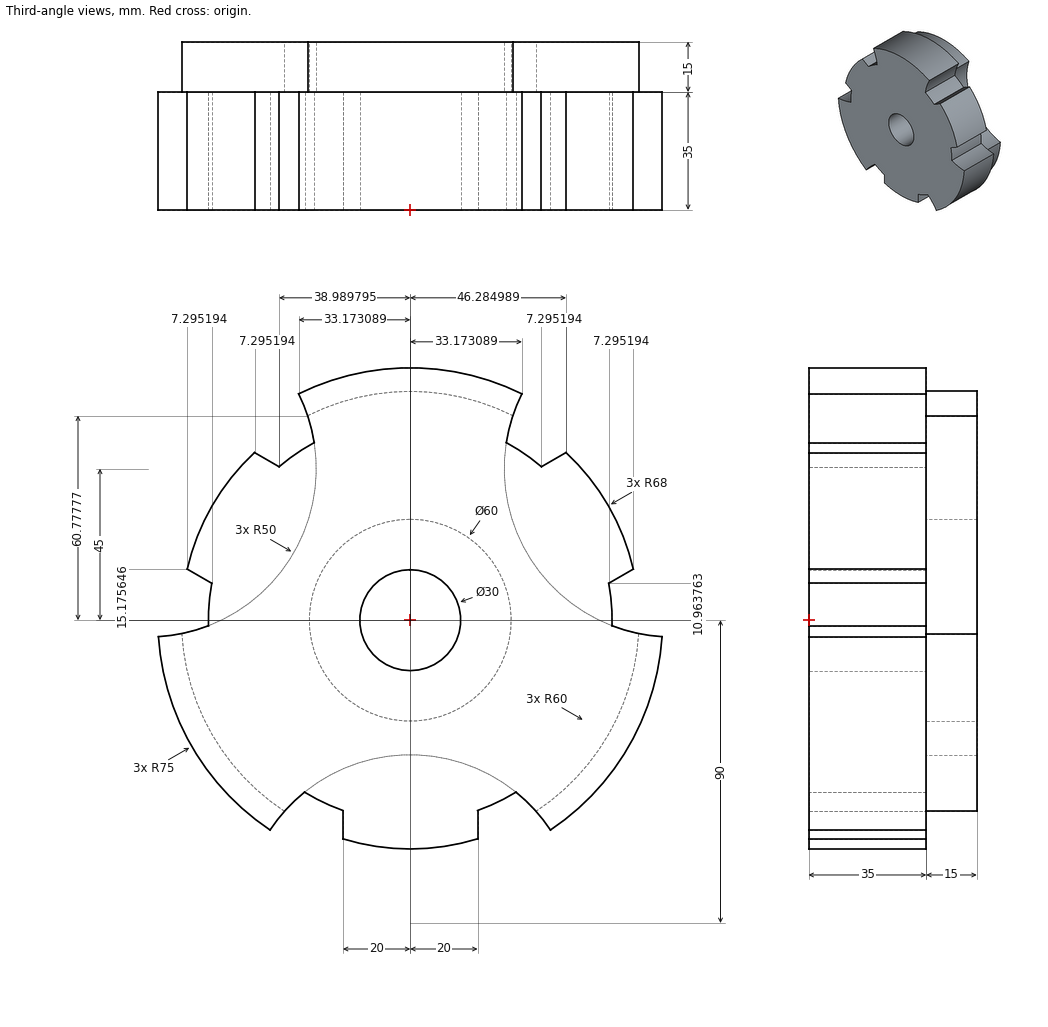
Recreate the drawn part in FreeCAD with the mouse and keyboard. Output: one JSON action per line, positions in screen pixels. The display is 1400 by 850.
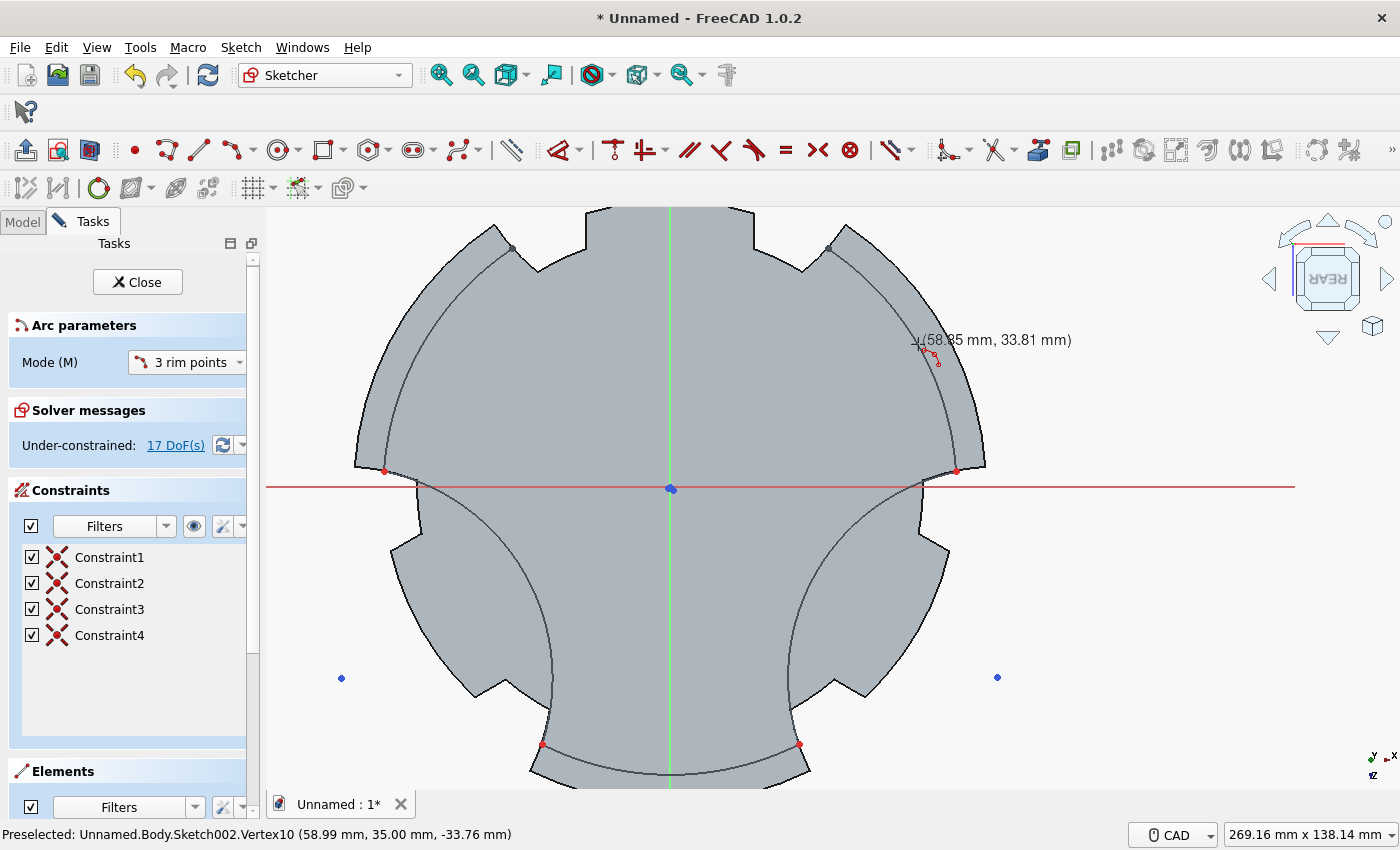
{"action": "left_click", "coordinate": [828, 249]}
{"action": "left_click", "coordinate": [512, 249]}
{"action": "left_click", "coordinate": [635, 316]}
{"action": "key", "text": "Escape"}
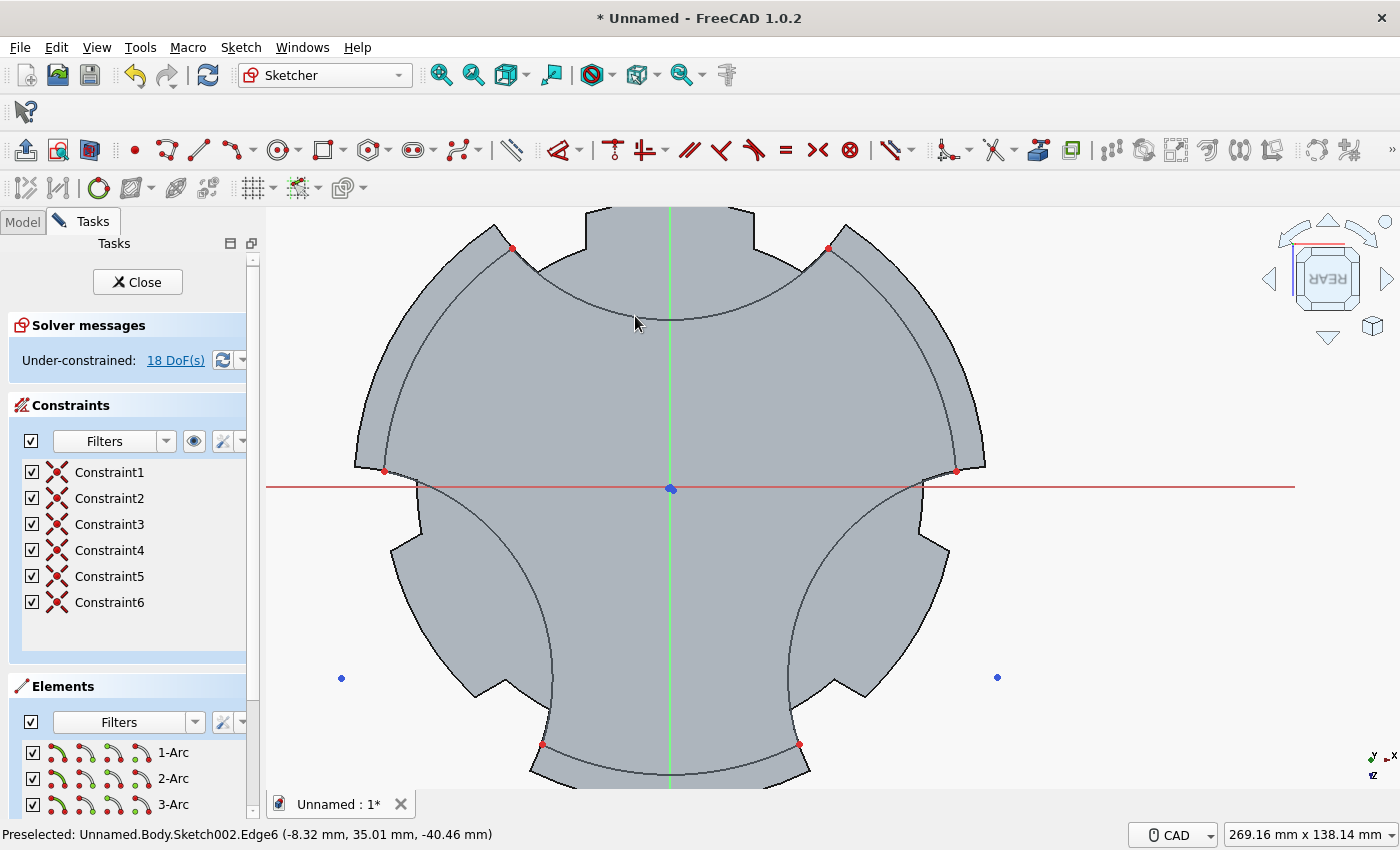
{"action": "left_click", "coordinate": [453, 302]}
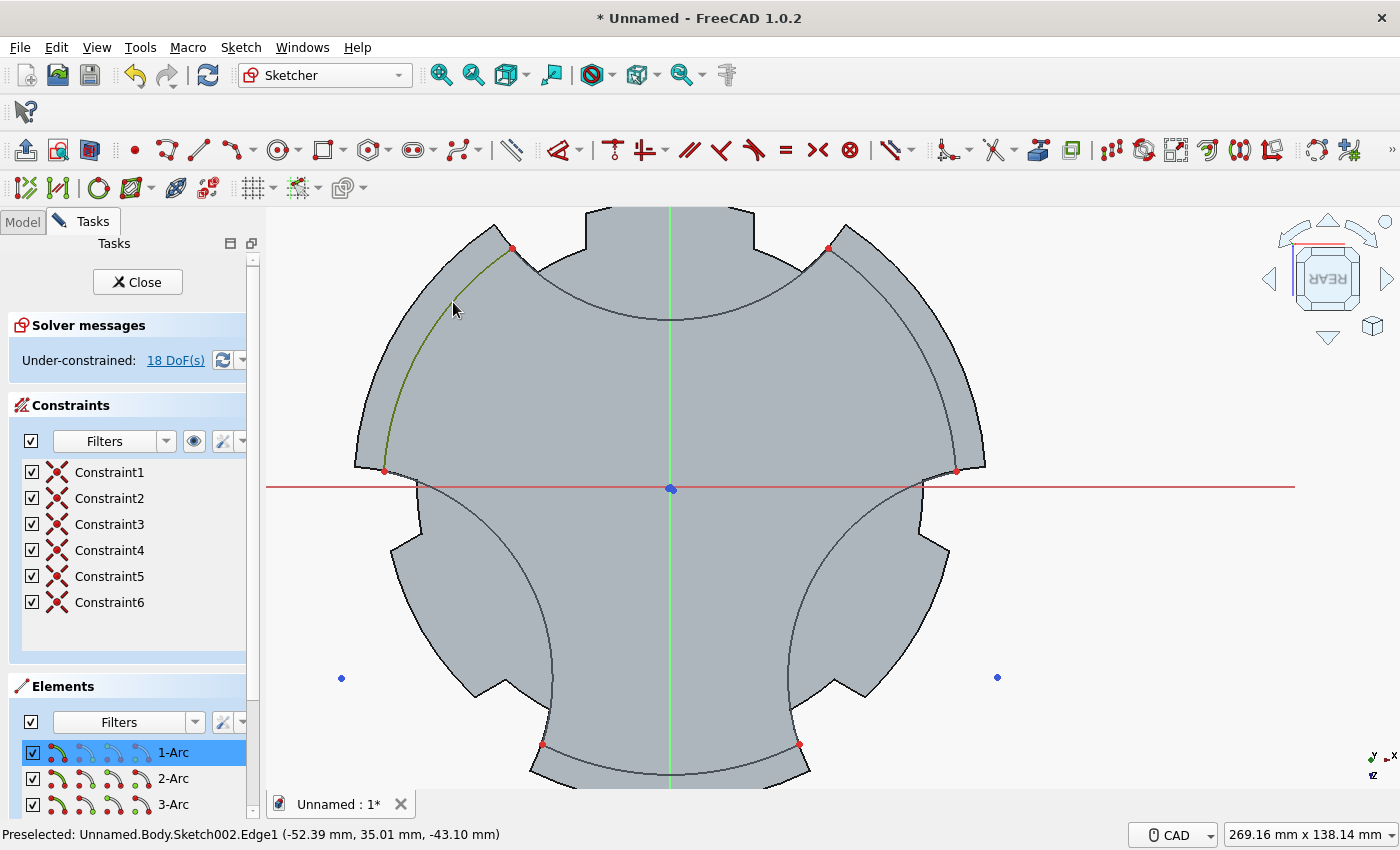
{"action": "scroll", "coordinate": [957, 471], "scroll_direction": "down", "scroll_amount": 2}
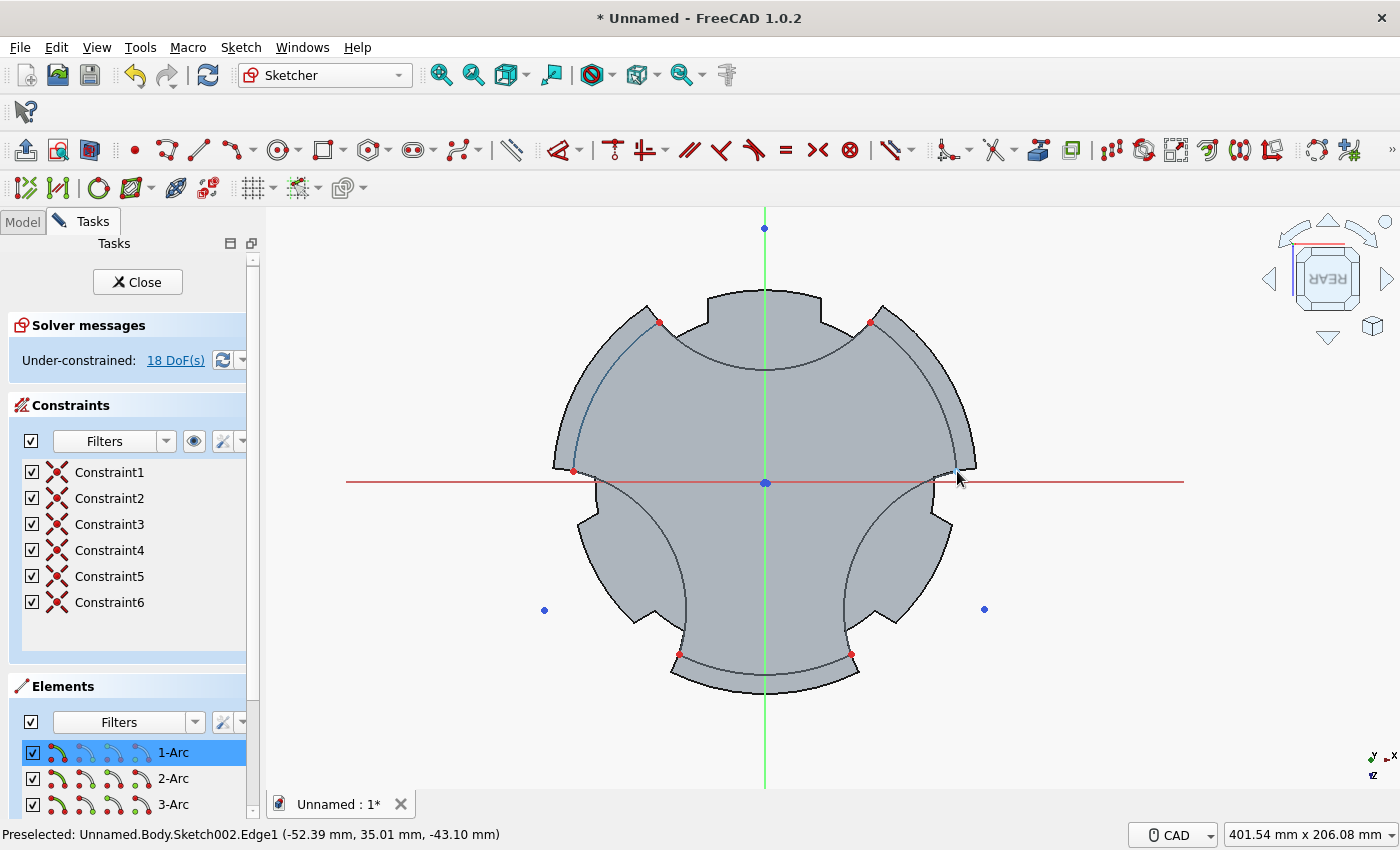
{"action": "left_click", "coordinate": [730, 672]}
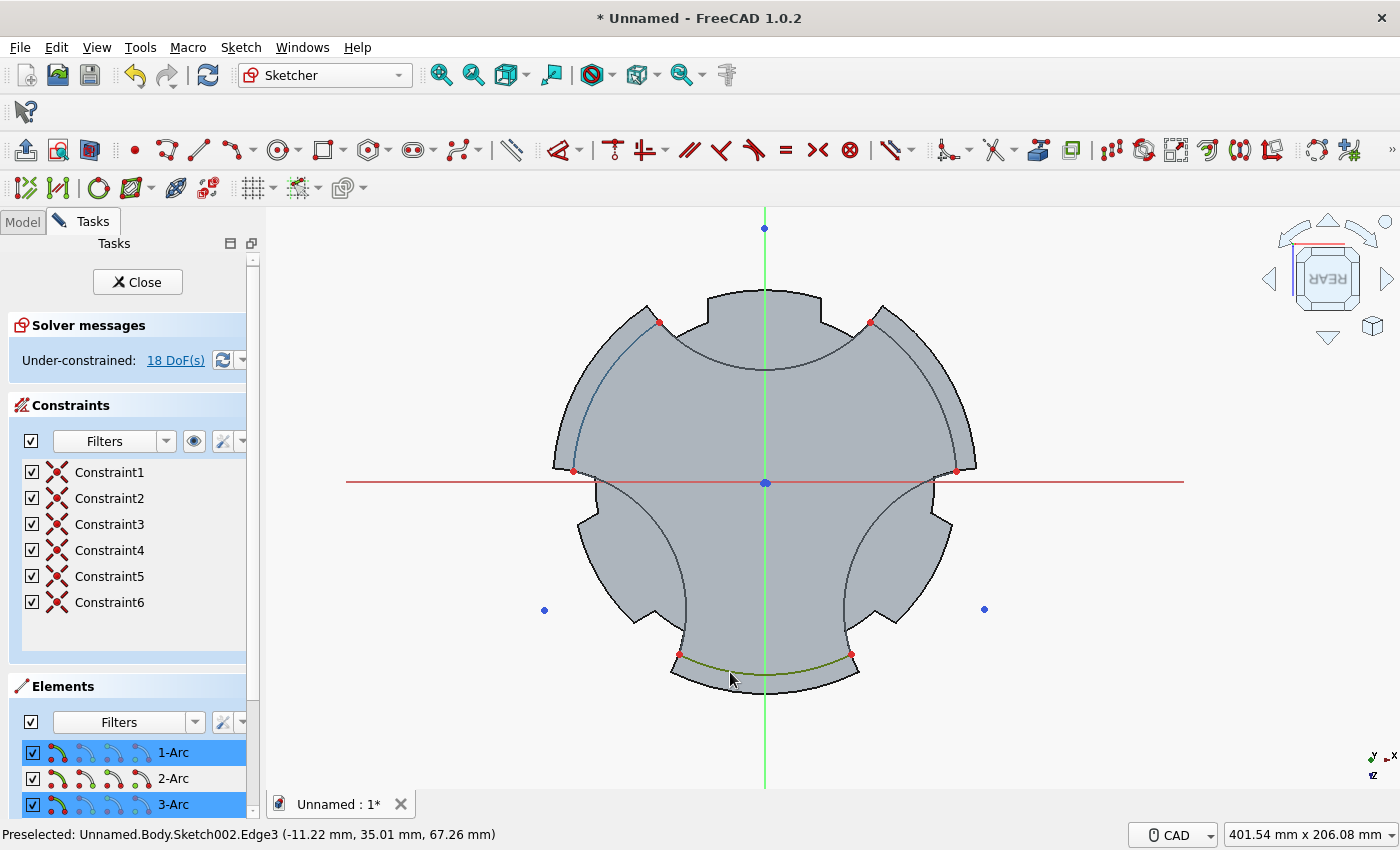
{"action": "left_click", "coordinate": [614, 150]}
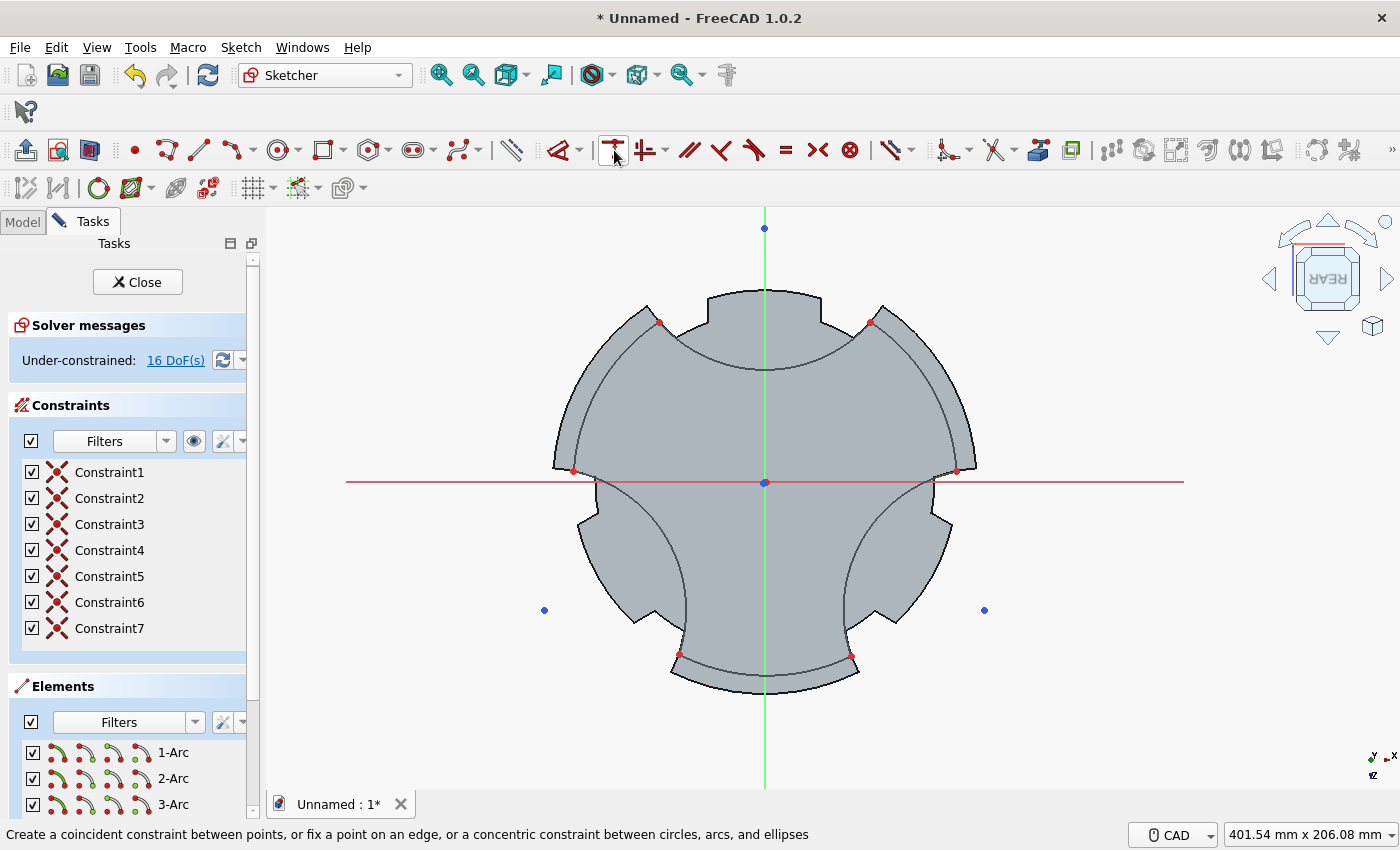
{"action": "left_click", "coordinate": [619, 358]}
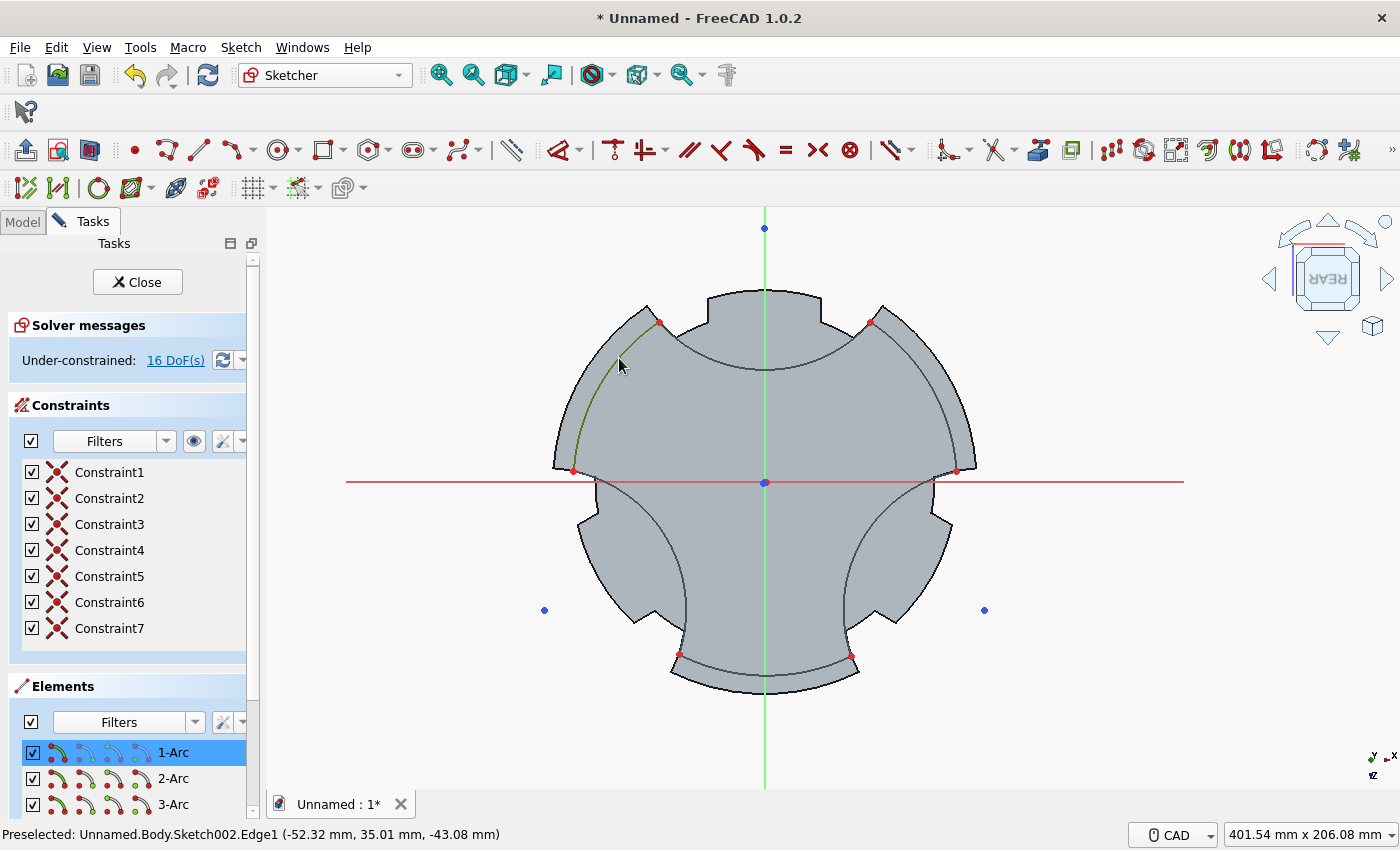
{"action": "left_click", "coordinate": [946, 419]}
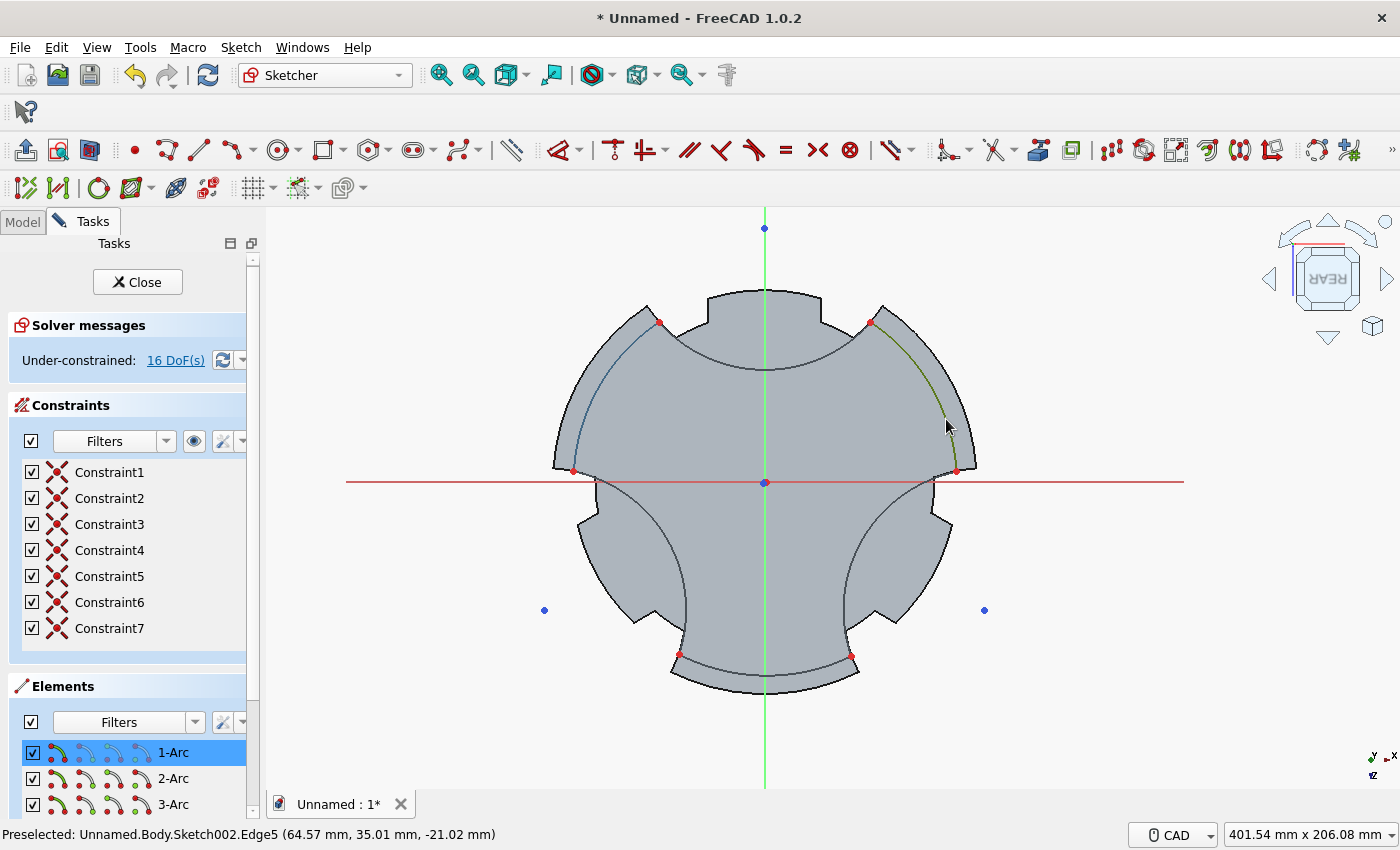
{"action": "left_click", "coordinate": [614, 150]}